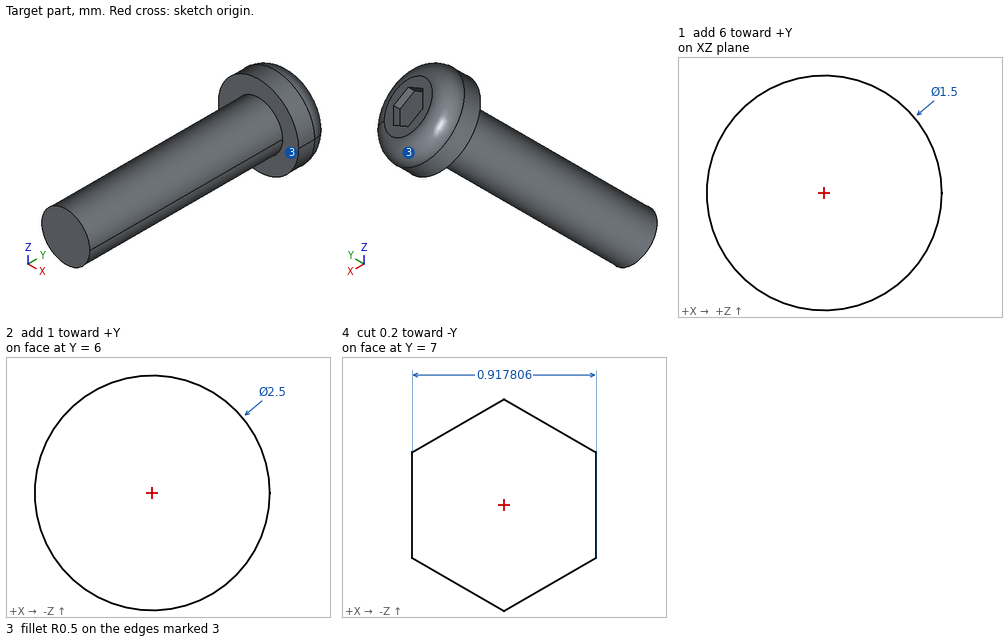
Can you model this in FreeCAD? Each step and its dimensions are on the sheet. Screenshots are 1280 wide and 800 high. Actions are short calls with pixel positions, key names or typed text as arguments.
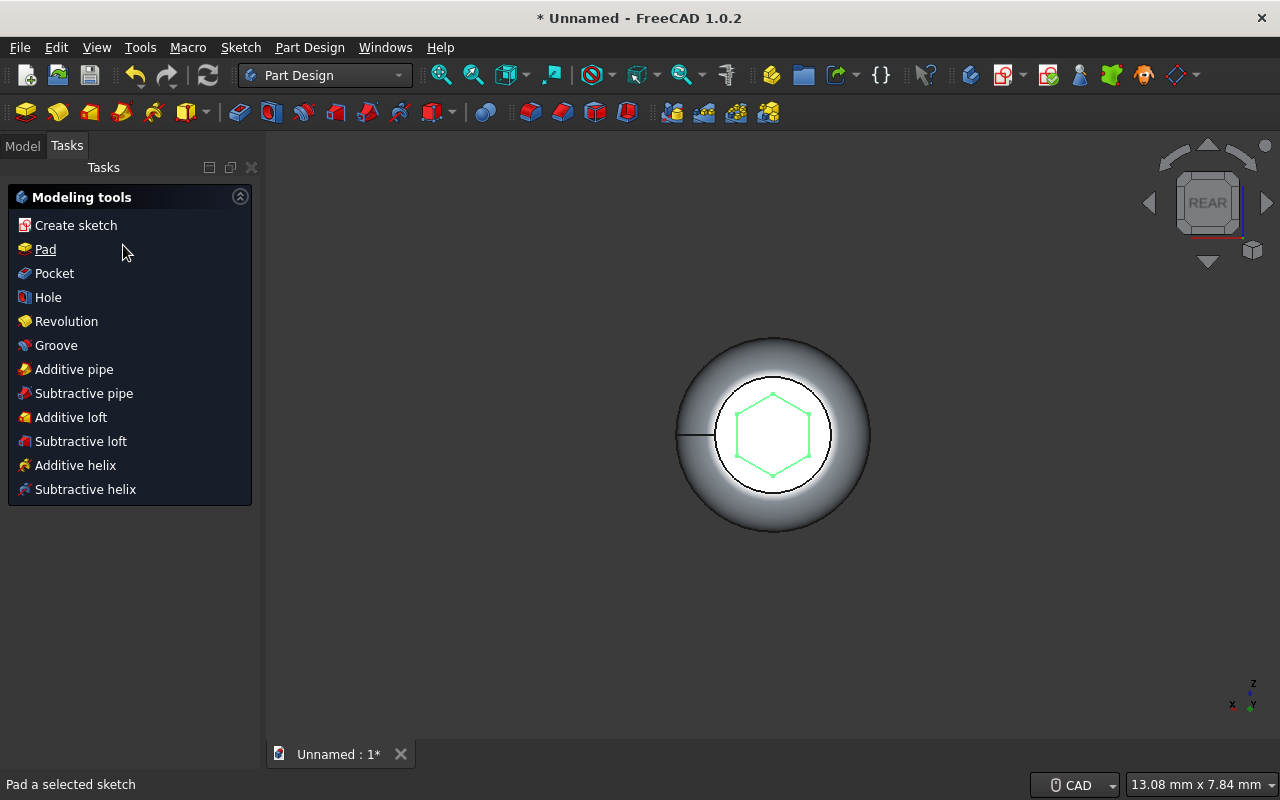
click(240, 112)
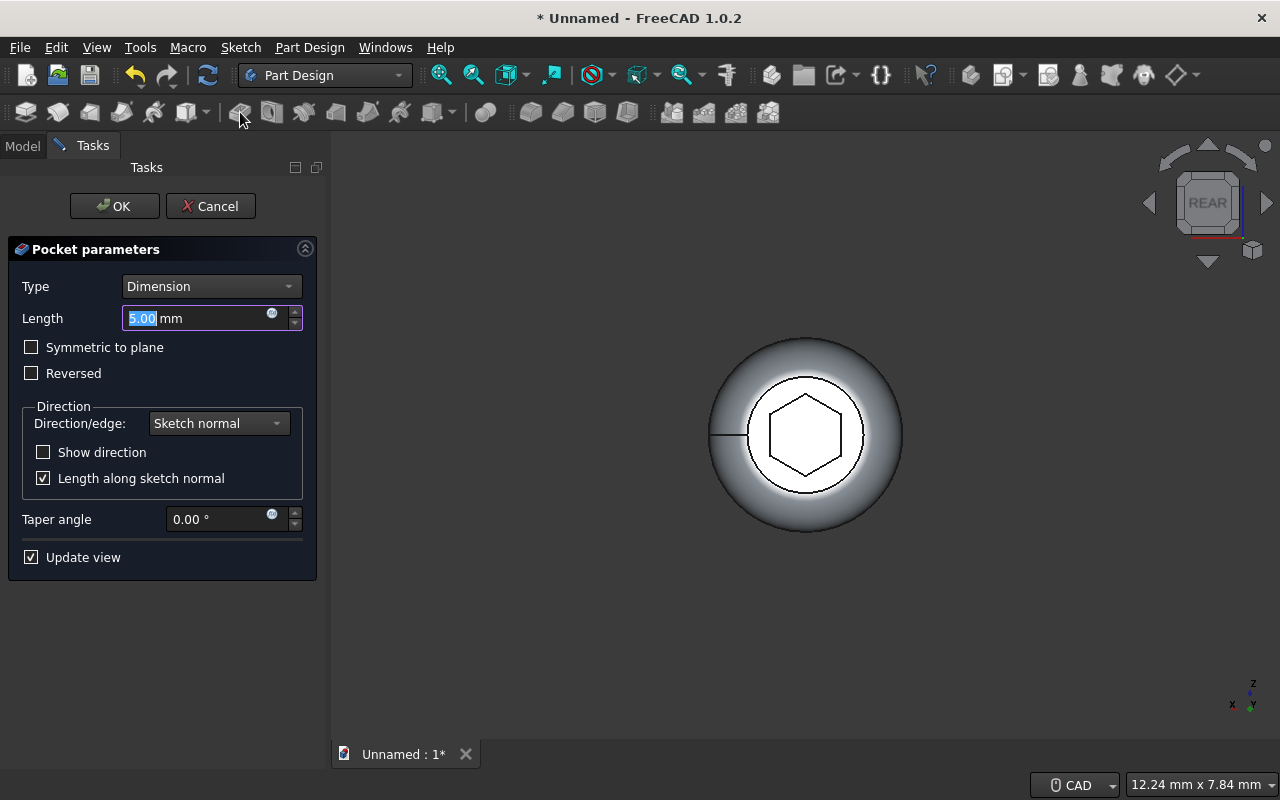
text(0.2)
key(Tab)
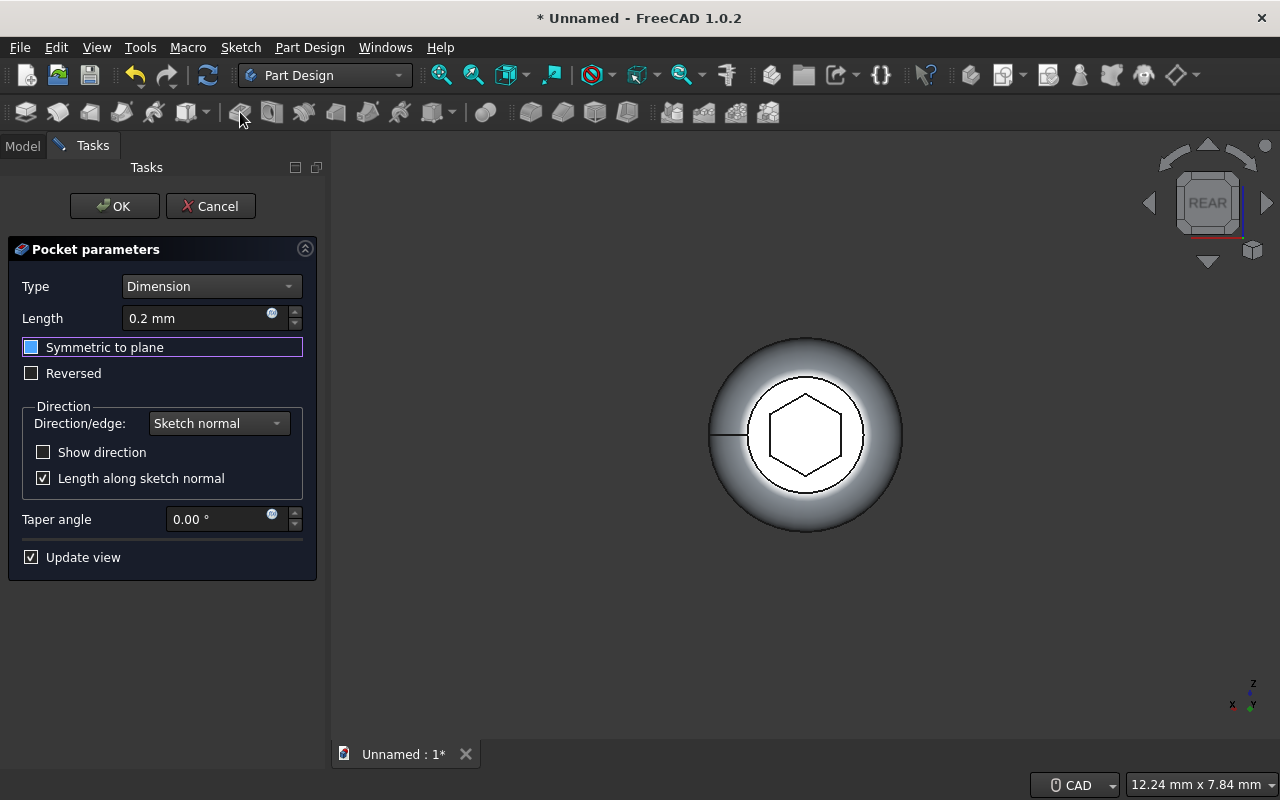
click(115, 206)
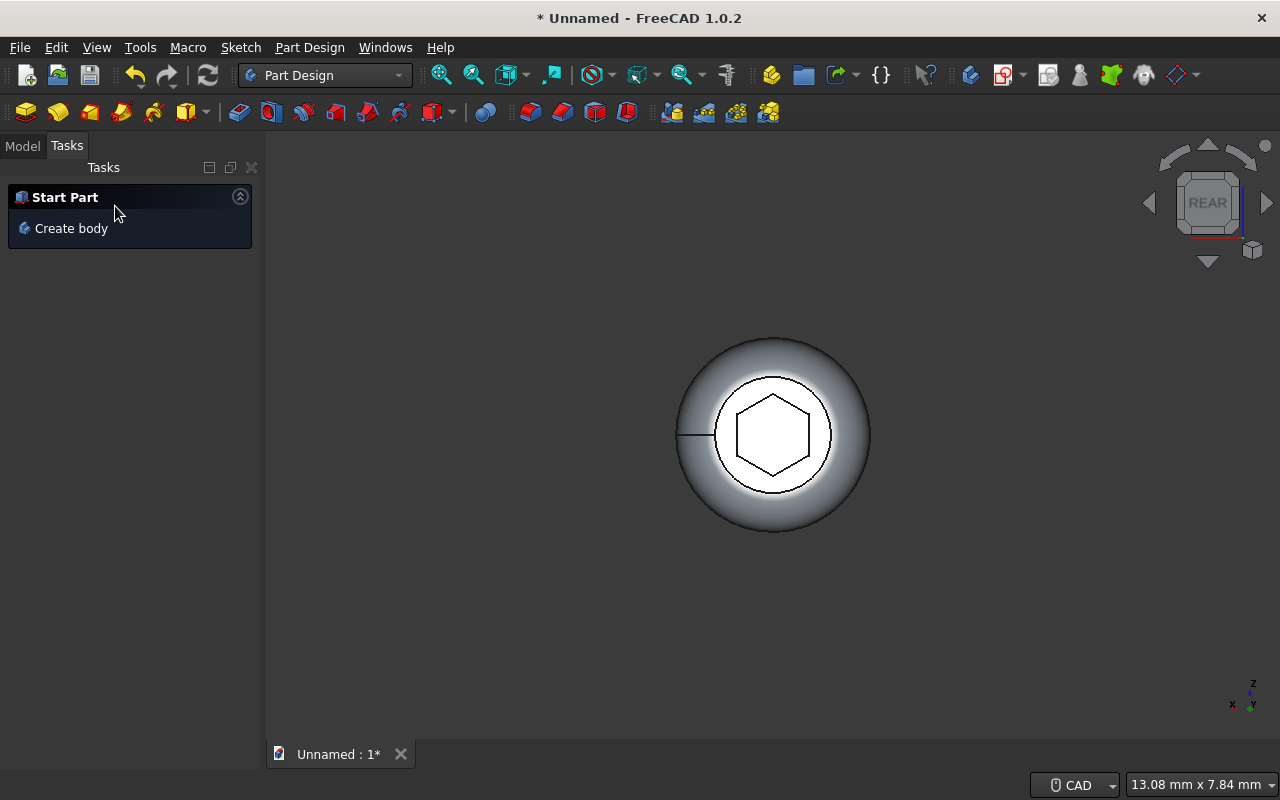
key(0)